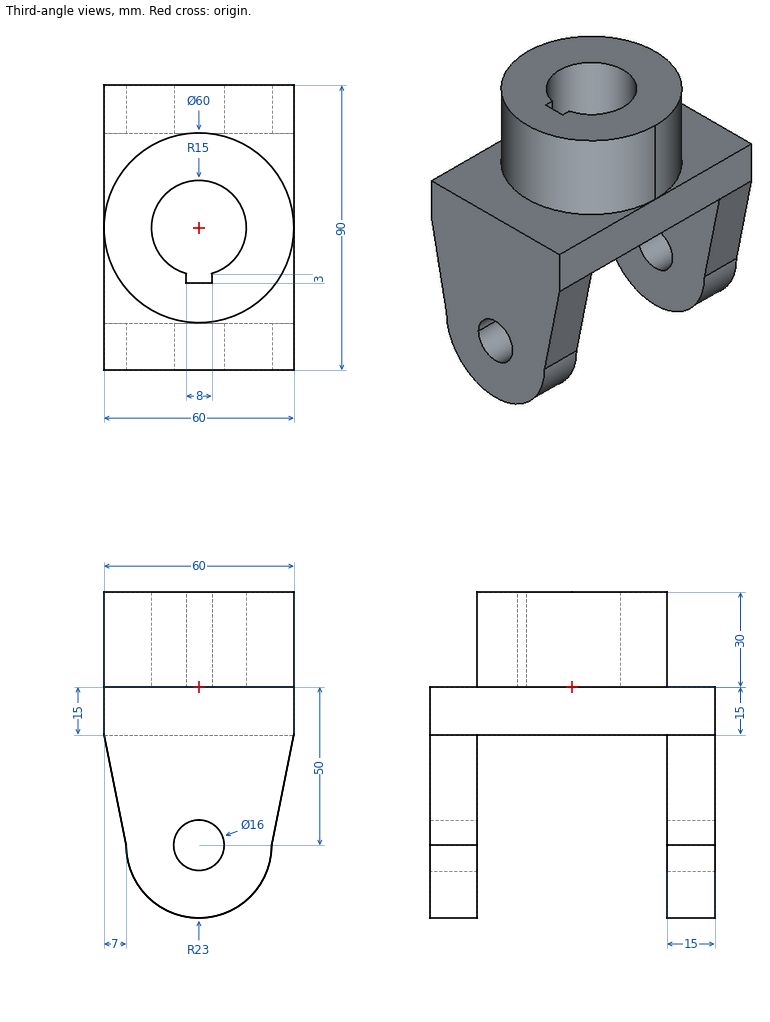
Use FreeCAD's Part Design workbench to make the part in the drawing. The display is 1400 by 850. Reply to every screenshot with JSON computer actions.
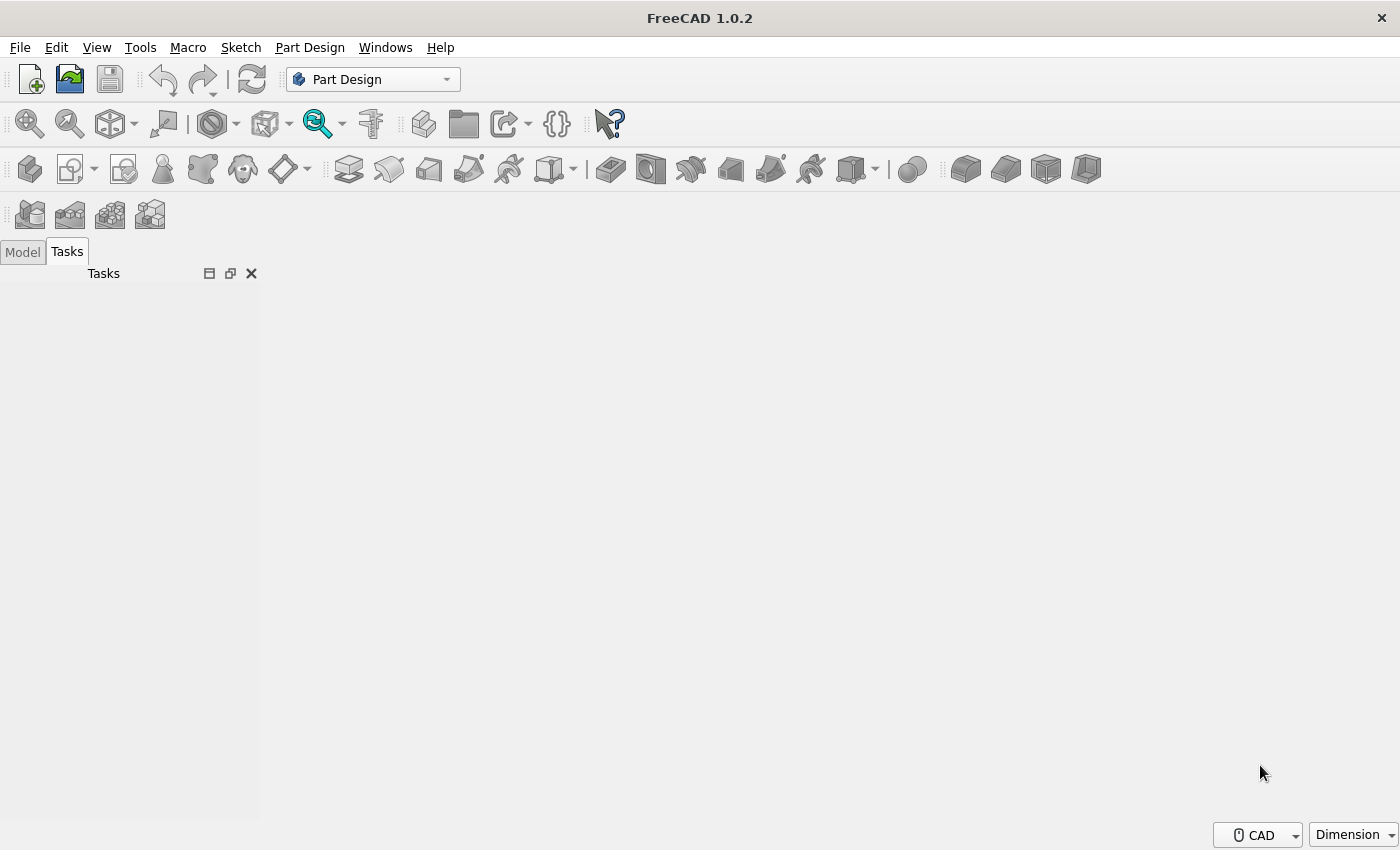
{"action": "left_click", "coordinate": [30, 80]}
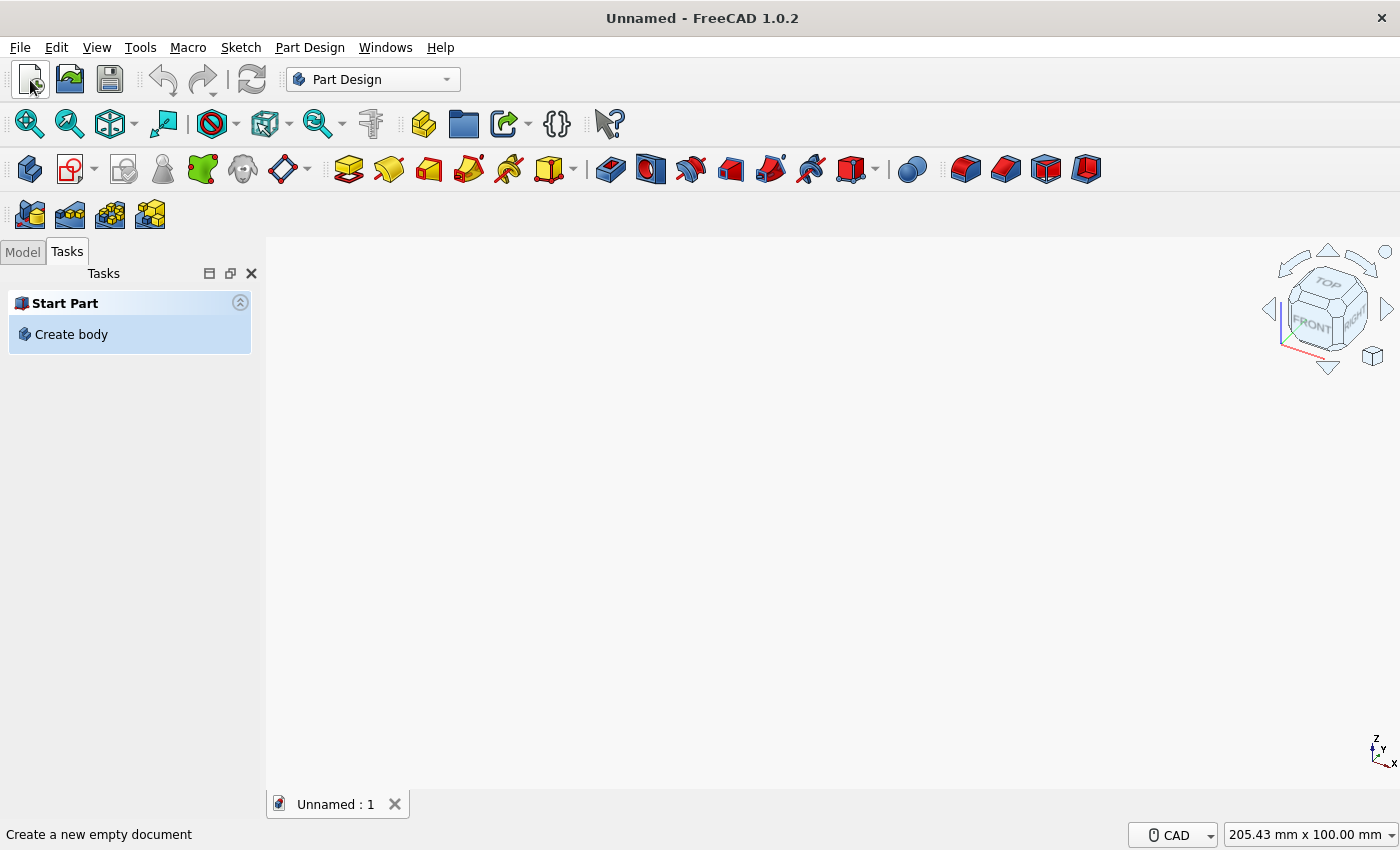
{"action": "left_click", "coordinate": [70, 170]}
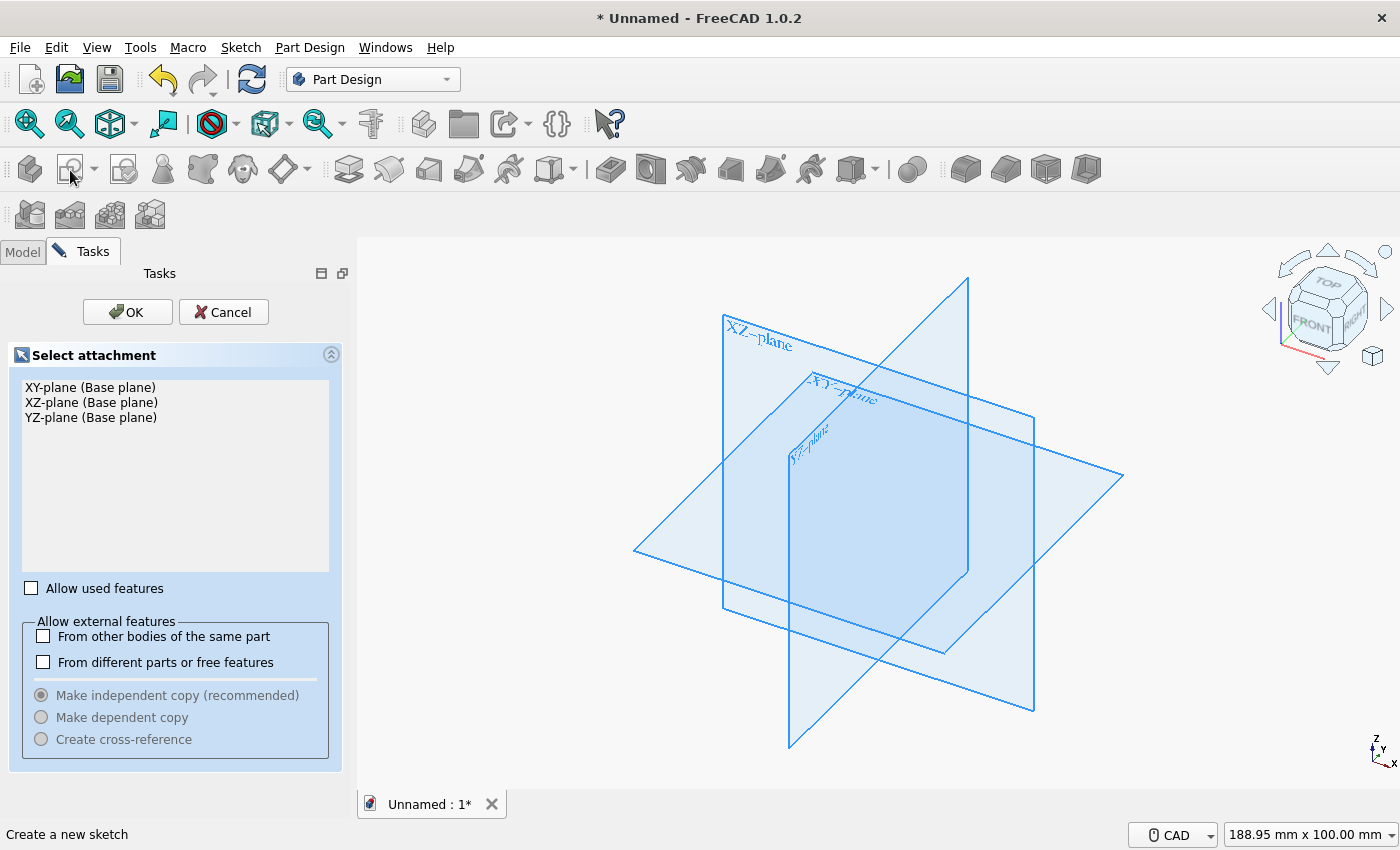
{"action": "left_click", "coordinate": [82, 388]}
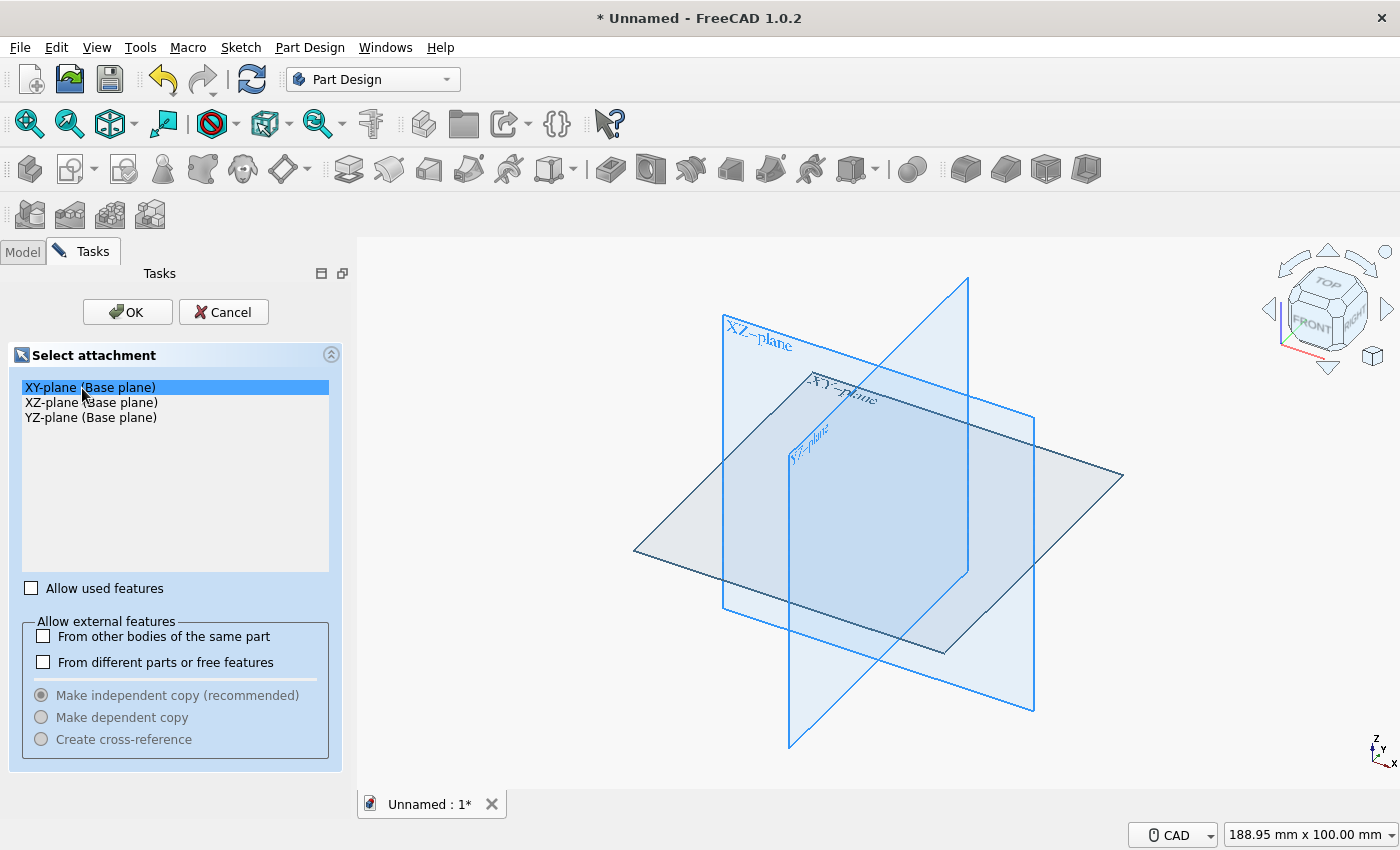
{"action": "left_click", "coordinate": [128, 312]}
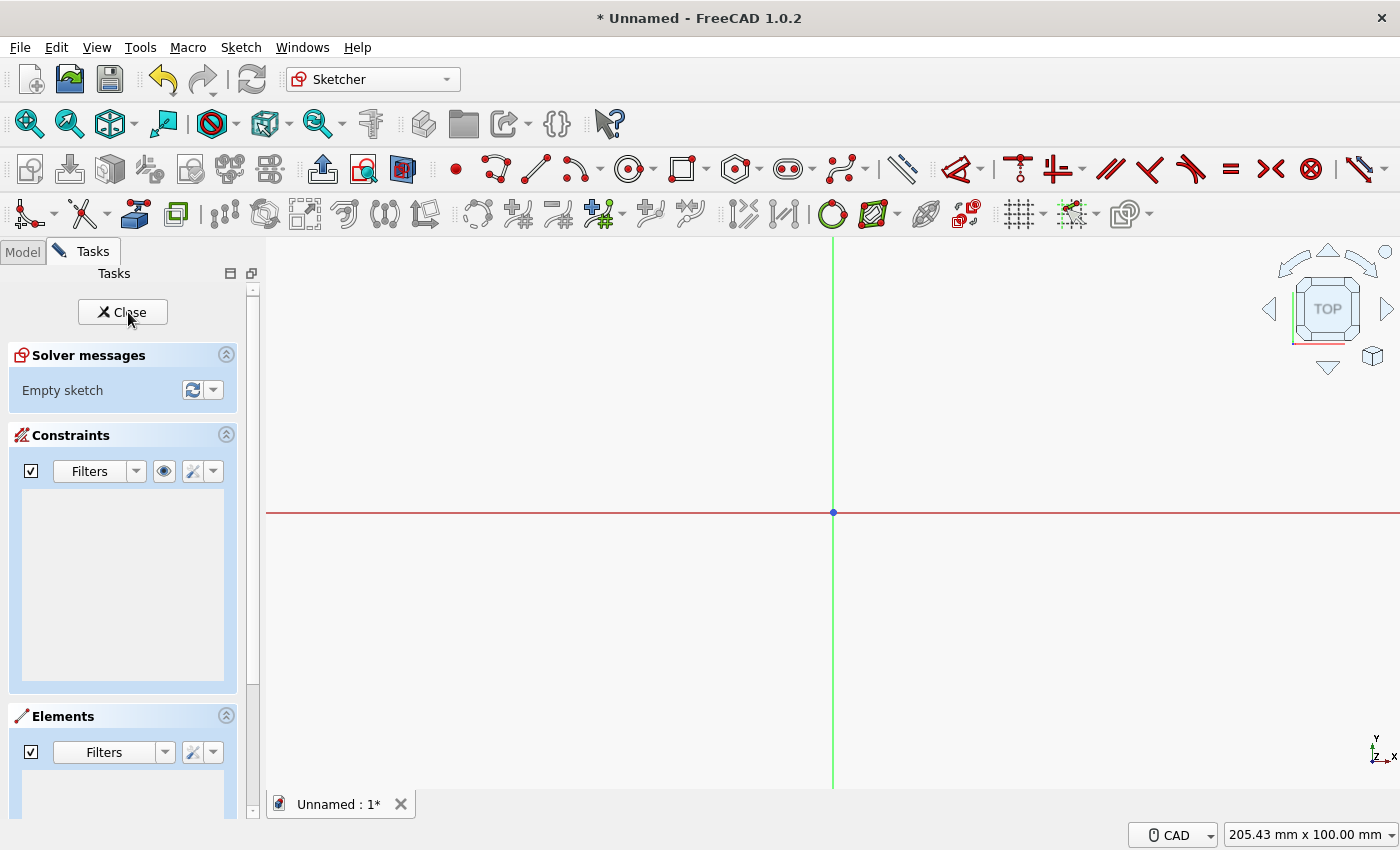
{"action": "scroll", "coordinate": [625, 513], "scroll_direction": "down", "scroll_amount": 2}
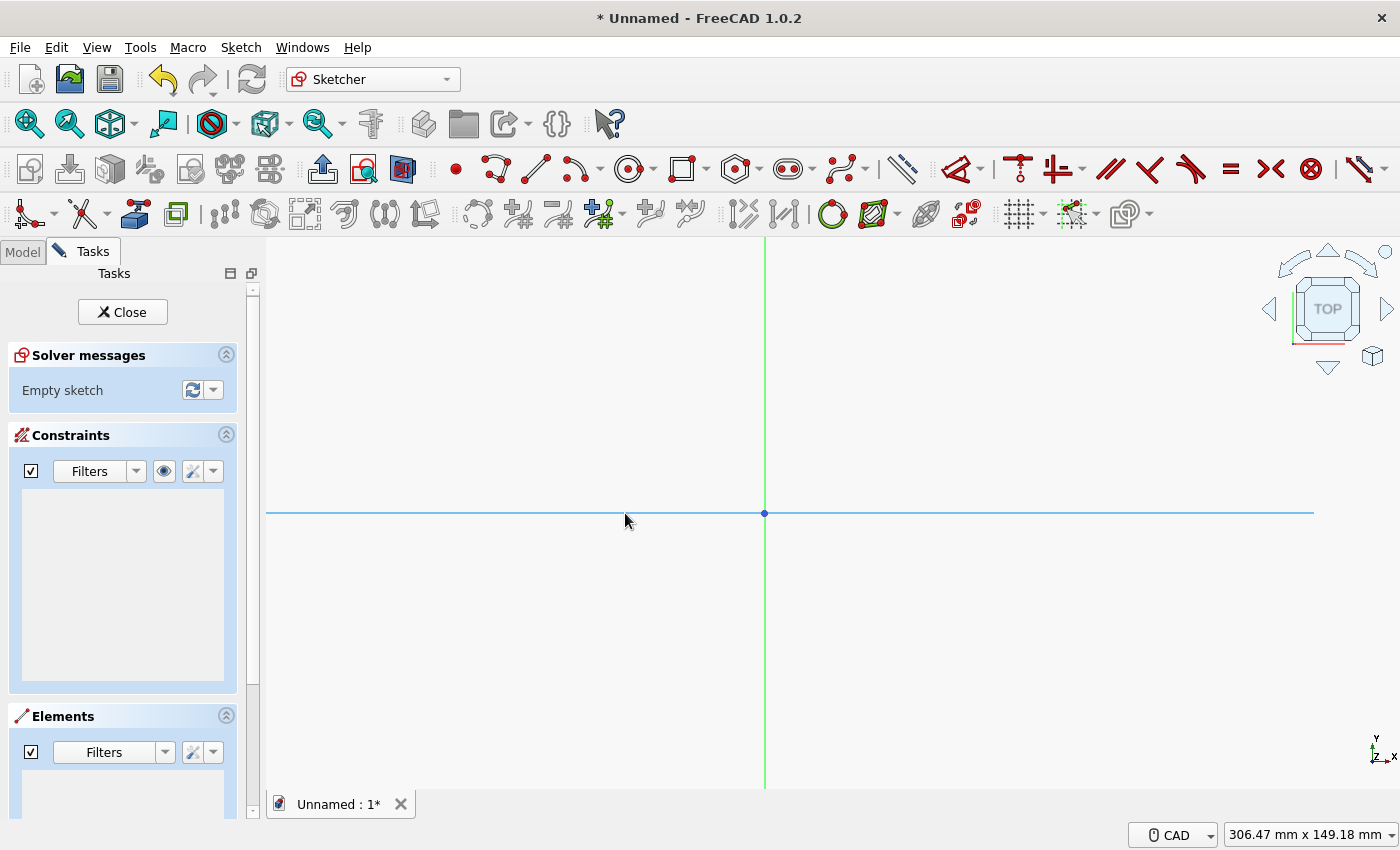
{"action": "key", "text": "g v"}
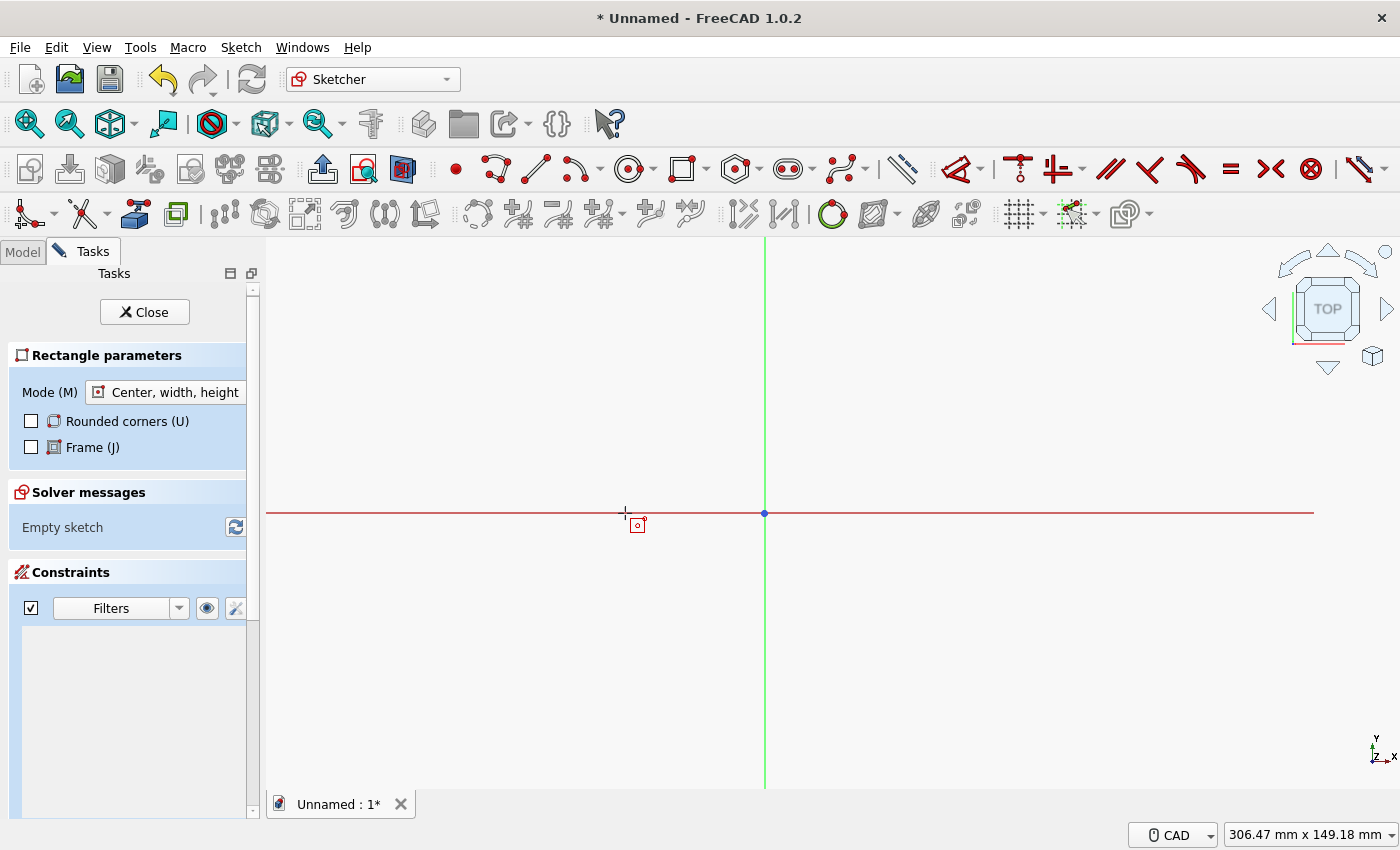
{"action": "left_click", "coordinate": [765, 513]}
{"action": "mouse_move", "coordinate": [876, 347]}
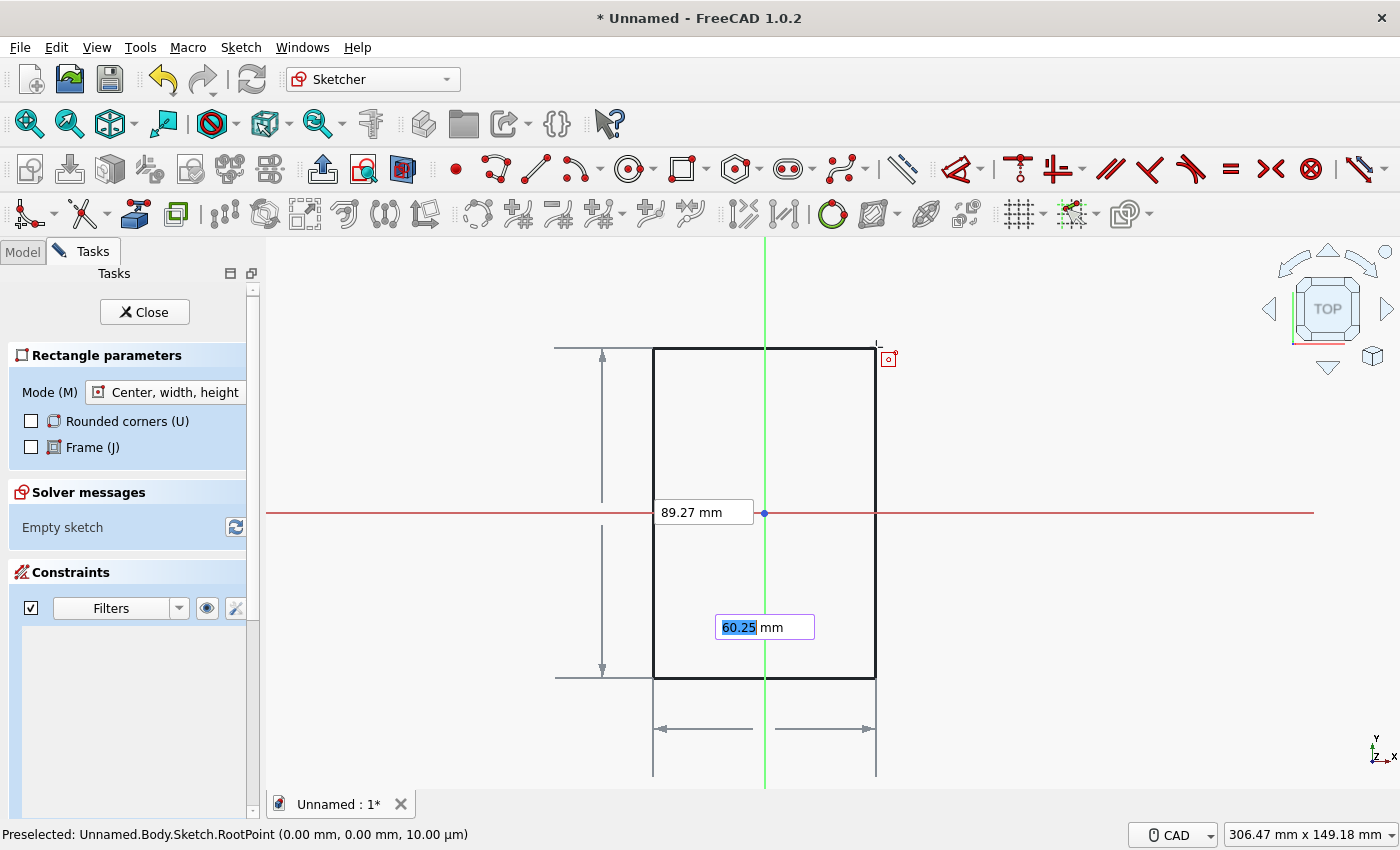
{"action": "type", "text": "60"}
{"action": "key", "text": "Tab"}
{"action": "type", "text": "90"}
{"action": "key", "text": "Return"}
{"action": "key", "text": "Escape"}